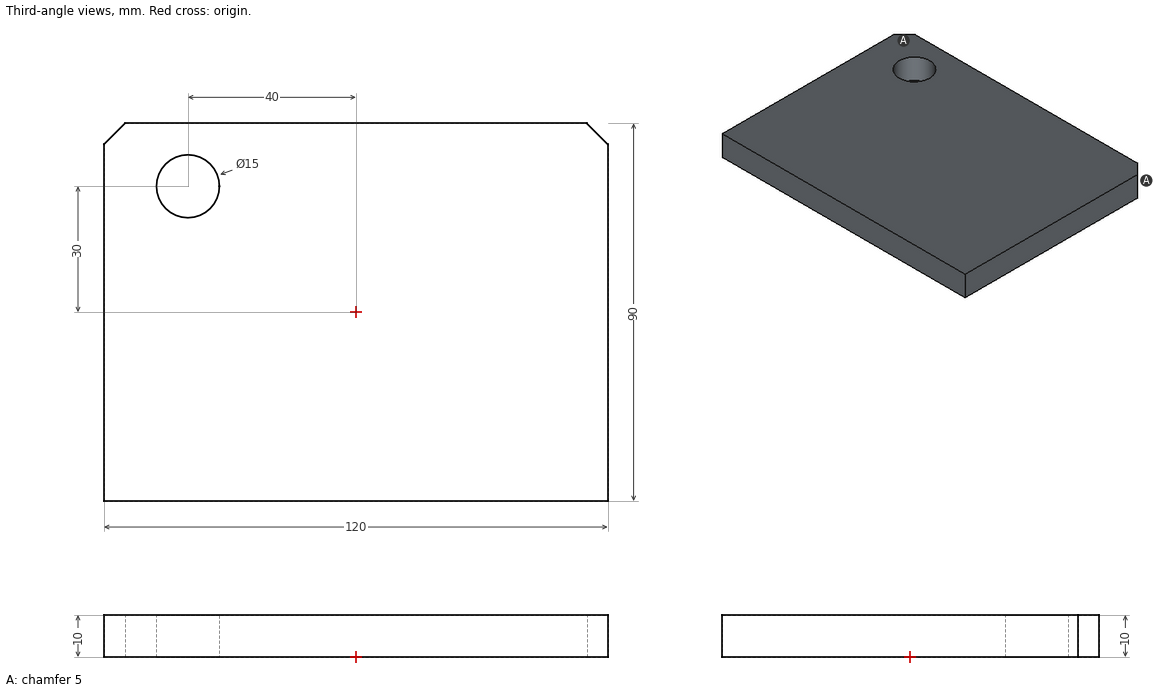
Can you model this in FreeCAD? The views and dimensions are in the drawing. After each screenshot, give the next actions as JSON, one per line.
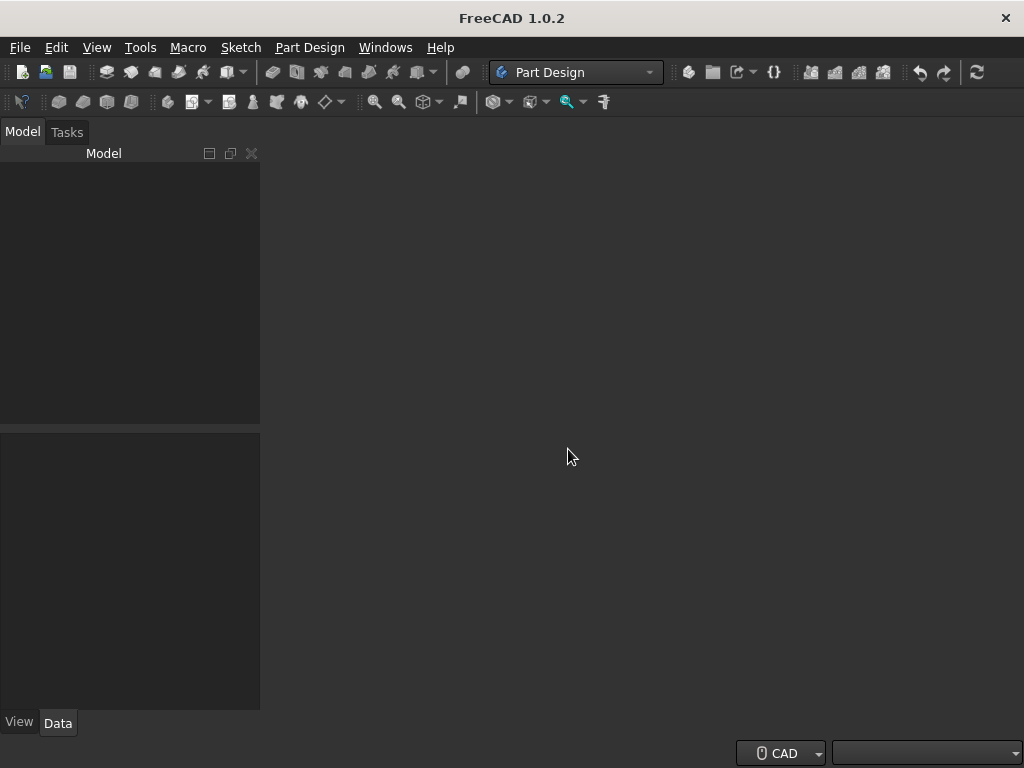
{"action": "left_click", "coordinate": [22, 72]}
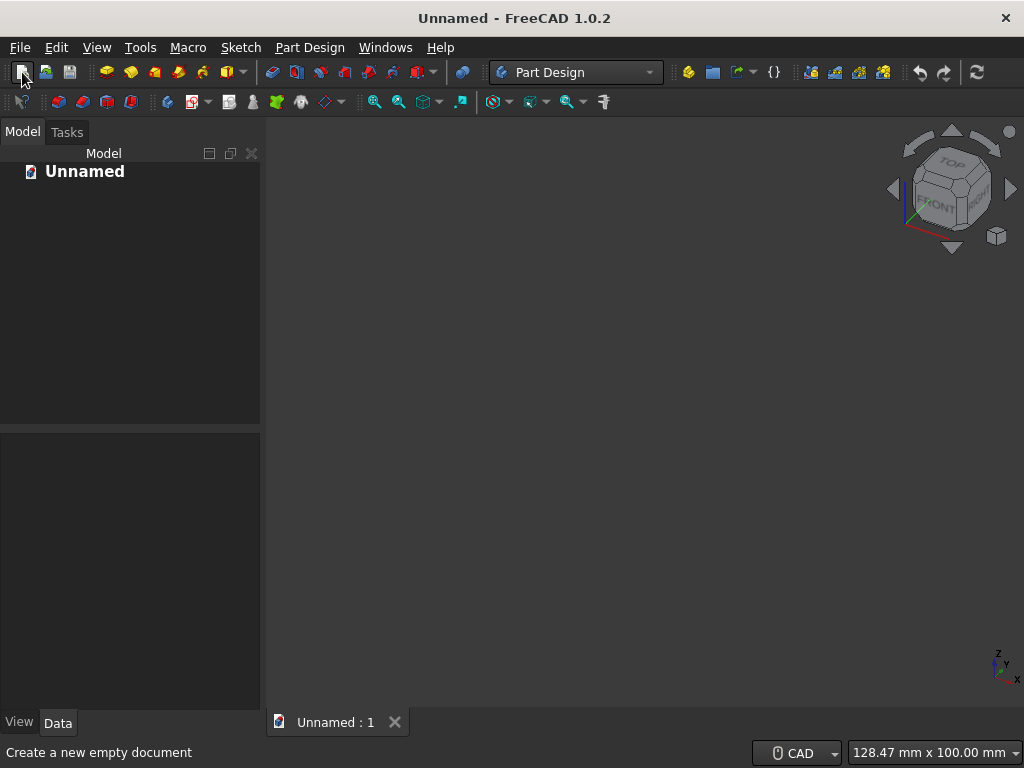
{"action": "left_click", "coordinate": [192, 102]}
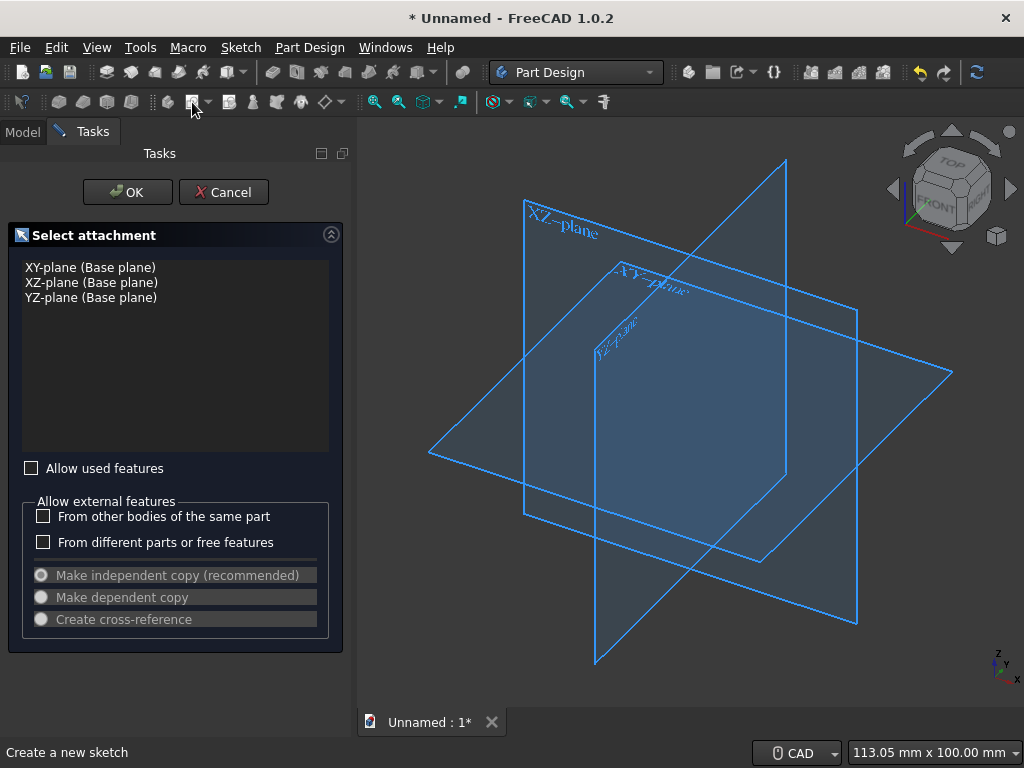
{"action": "left_click", "coordinate": [82, 268]}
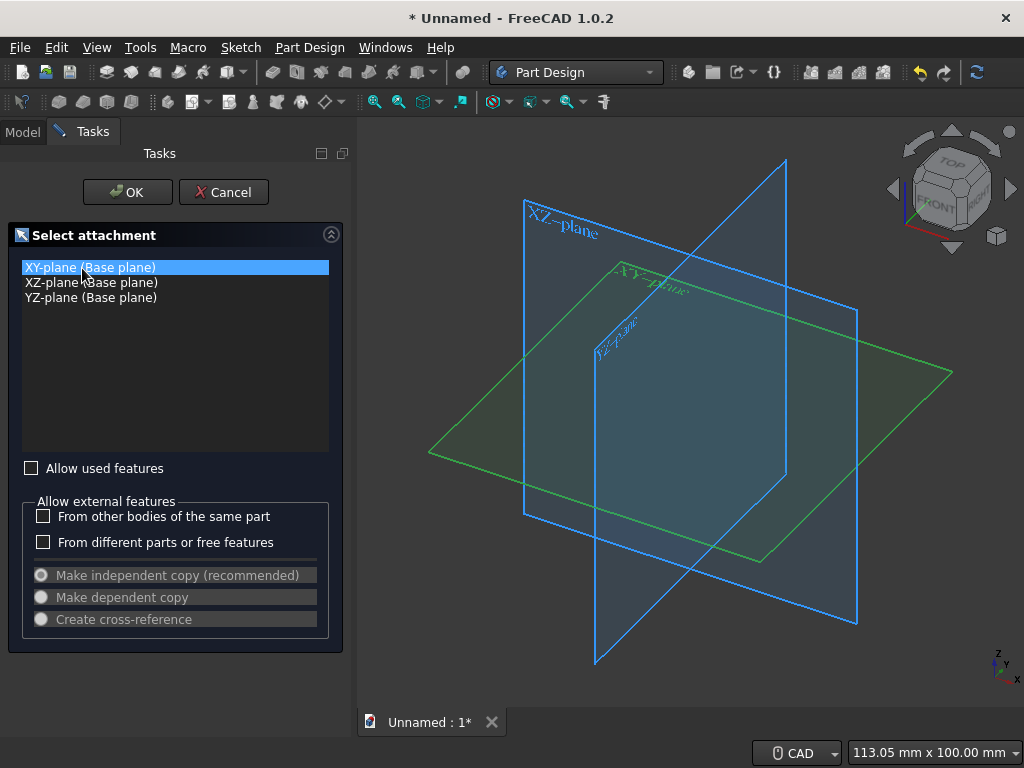
{"action": "left_click", "coordinate": [128, 192]}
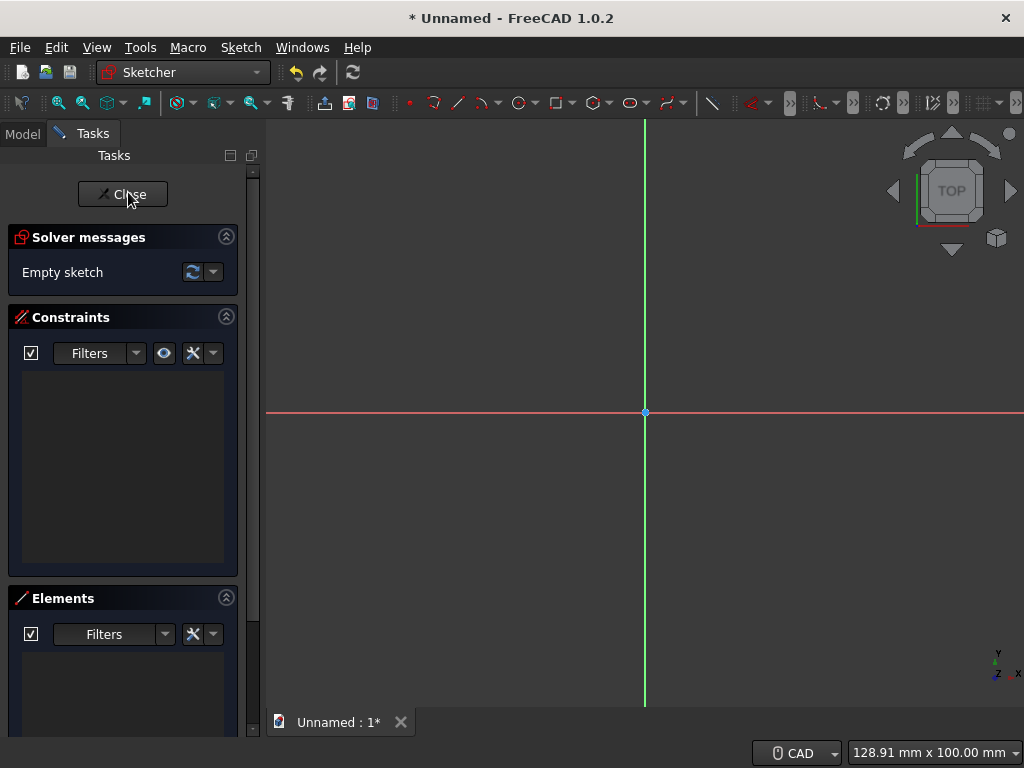
{"action": "scroll", "coordinate": [493, 413], "scroll_direction": "down", "scroll_amount": 3}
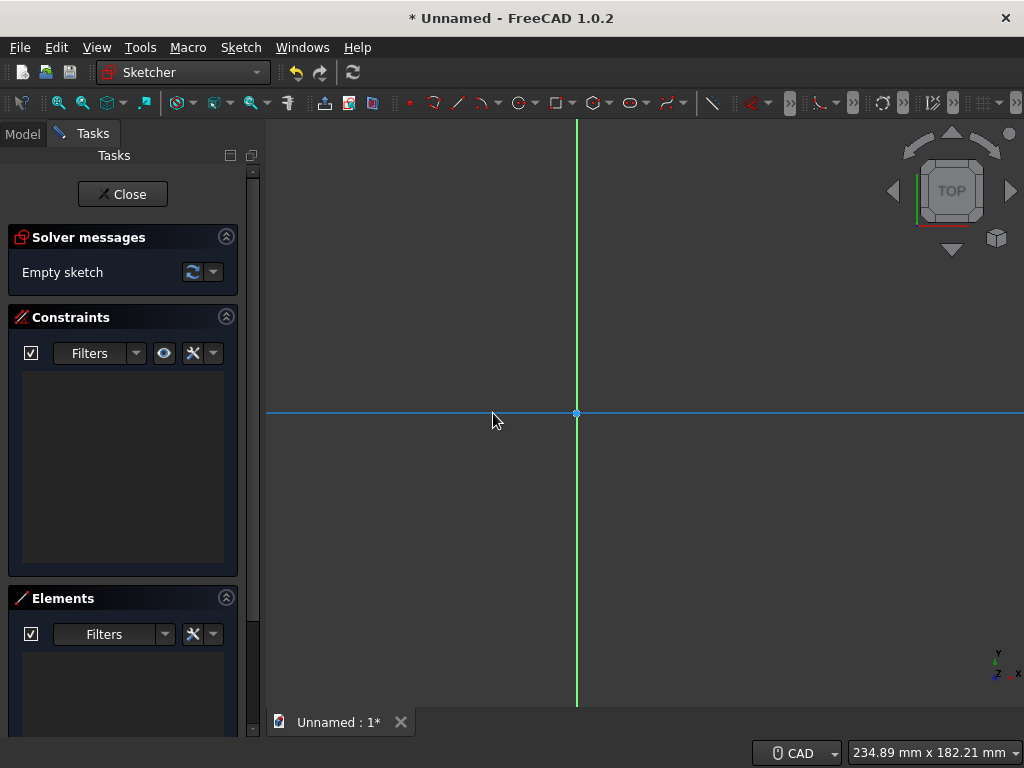
{"action": "left_click", "coordinate": [574, 104]}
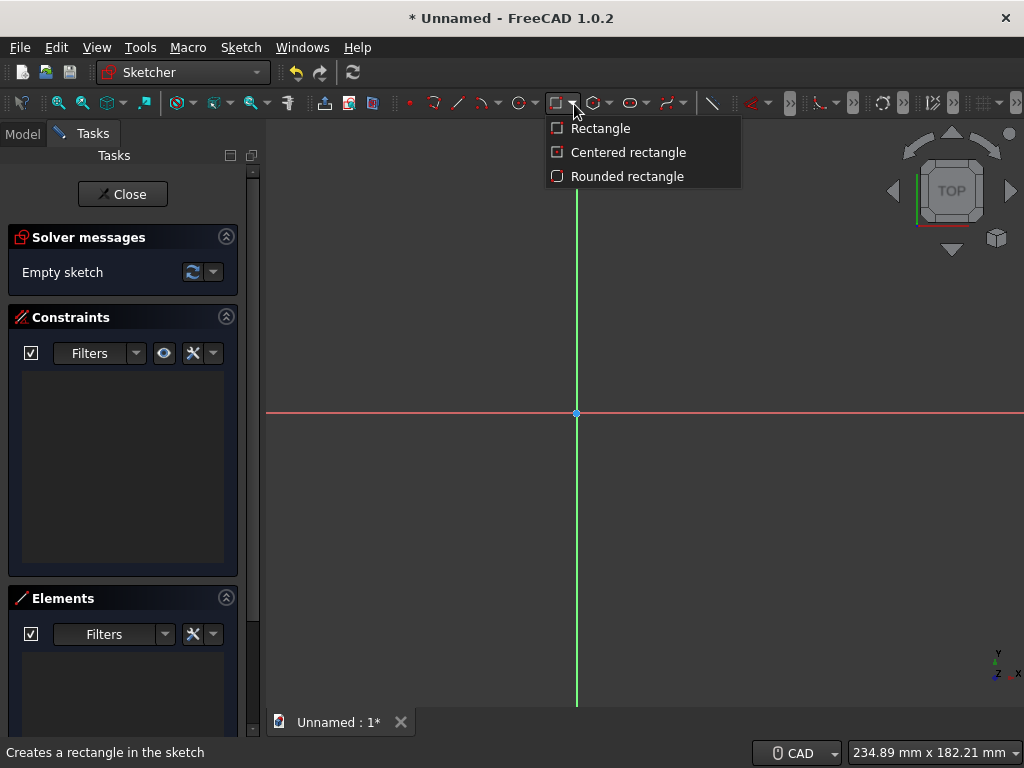
{"action": "left_click", "coordinate": [644, 152]}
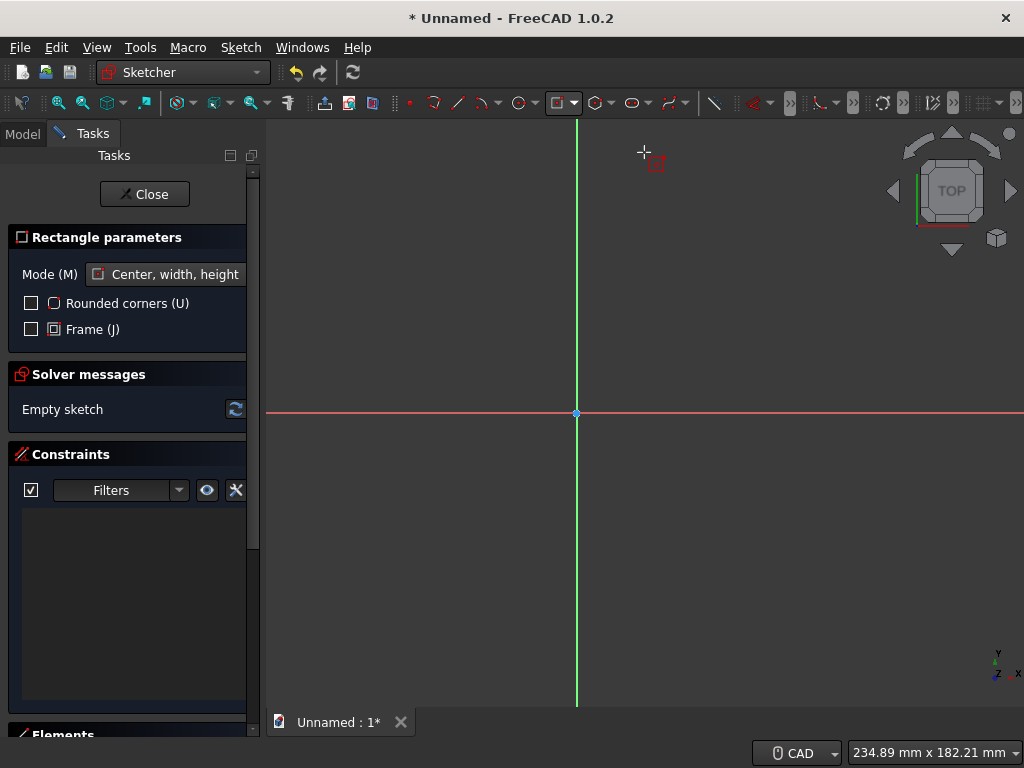
{"action": "left_click", "coordinate": [577, 413]}
{"action": "left_click", "coordinate": [770, 268]}
{"action": "key", "text": "Escape"}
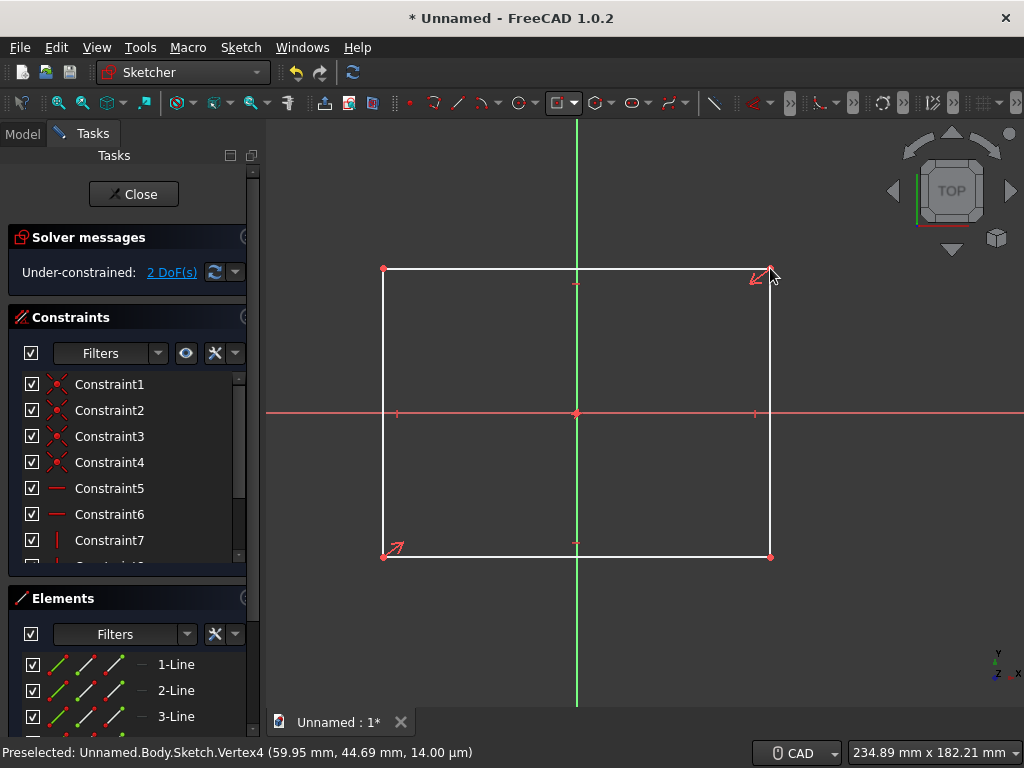
{"action": "left_click", "coordinate": [754, 104]}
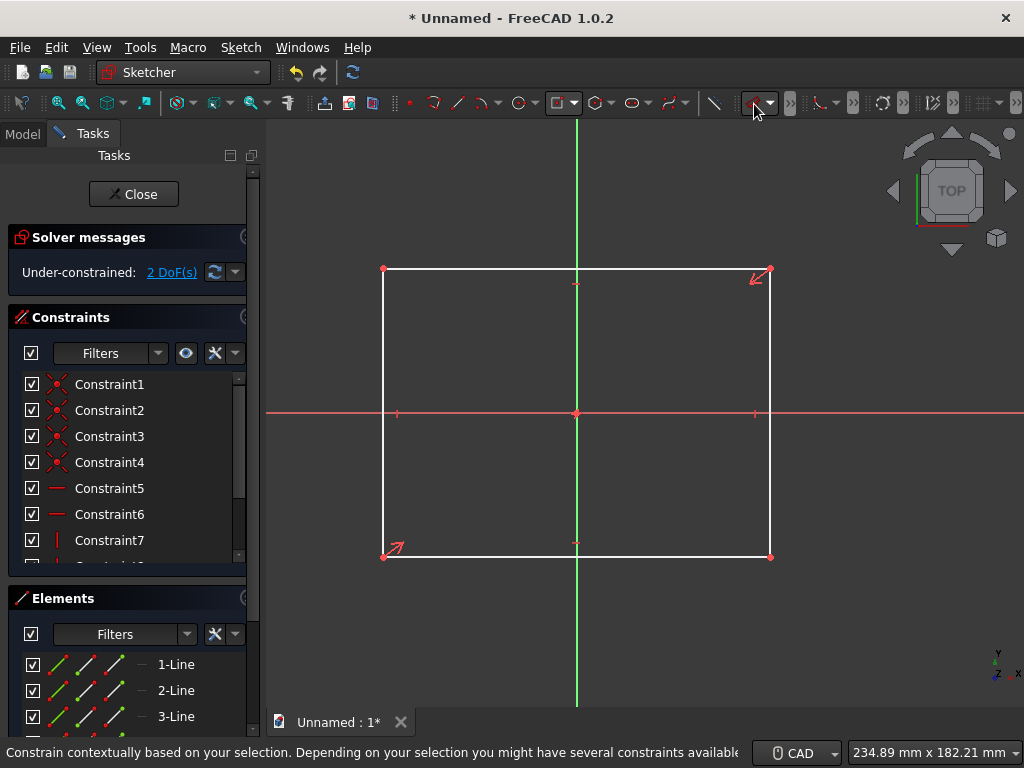
{"action": "left_click", "coordinate": [770, 471]}
{"action": "left_click", "coordinate": [804, 347]}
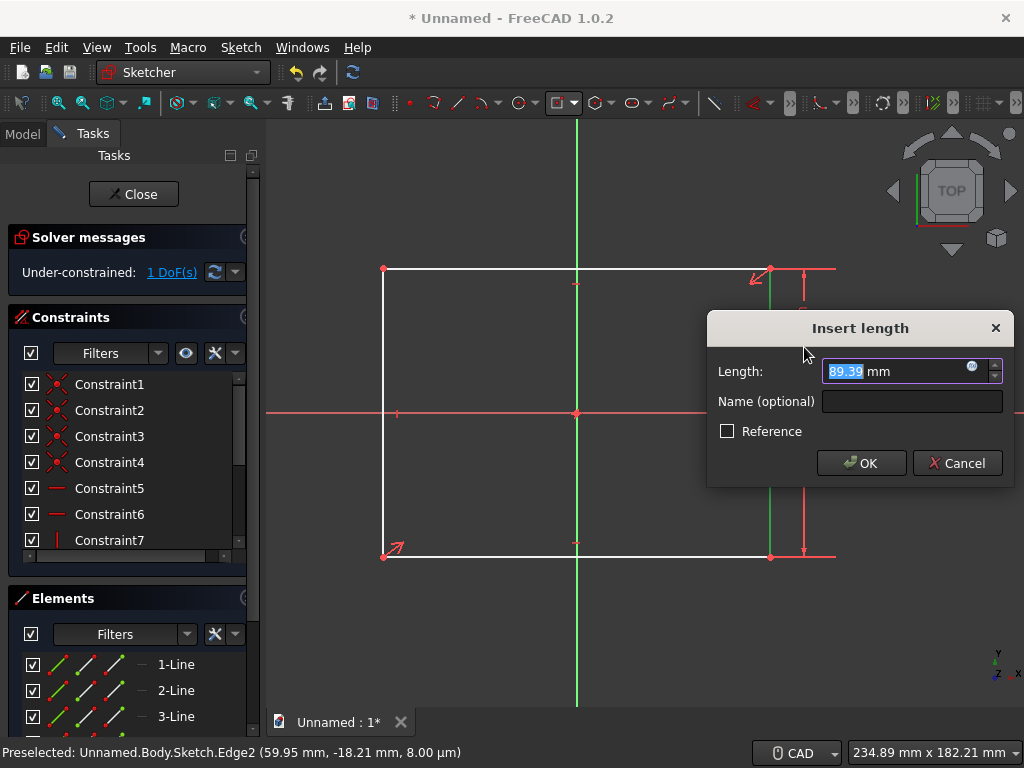
{"action": "type", "text": "90"}
{"action": "key", "text": "Return"}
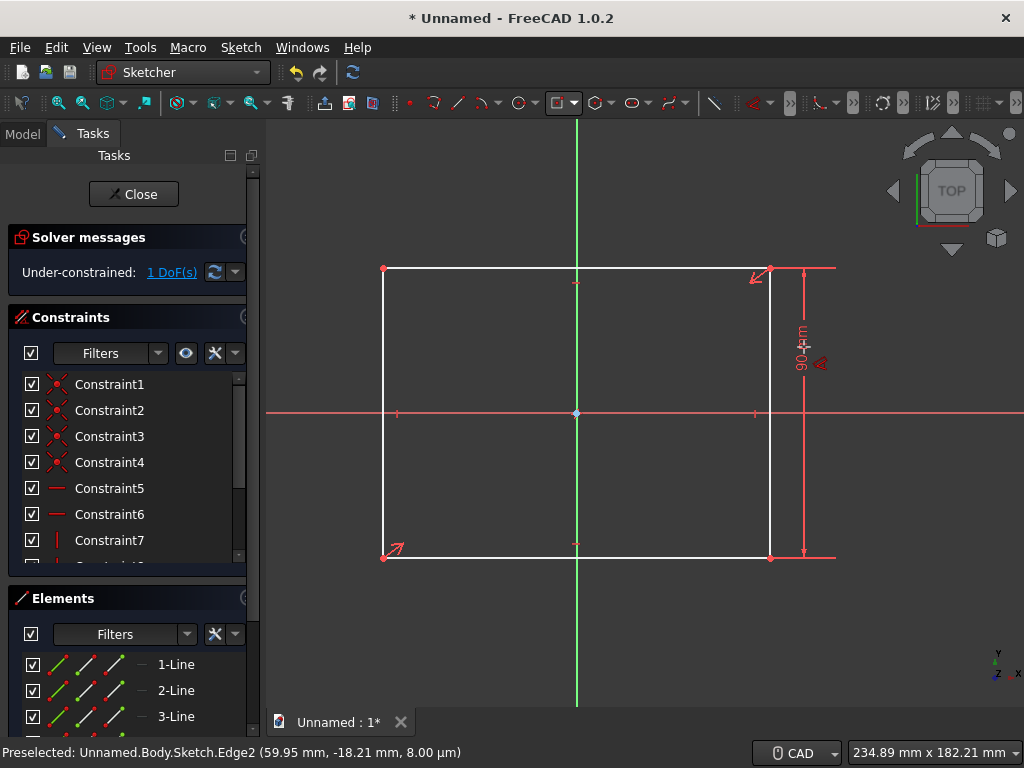
{"action": "left_click", "coordinate": [499, 558]}
{"action": "left_click", "coordinate": [488, 592]}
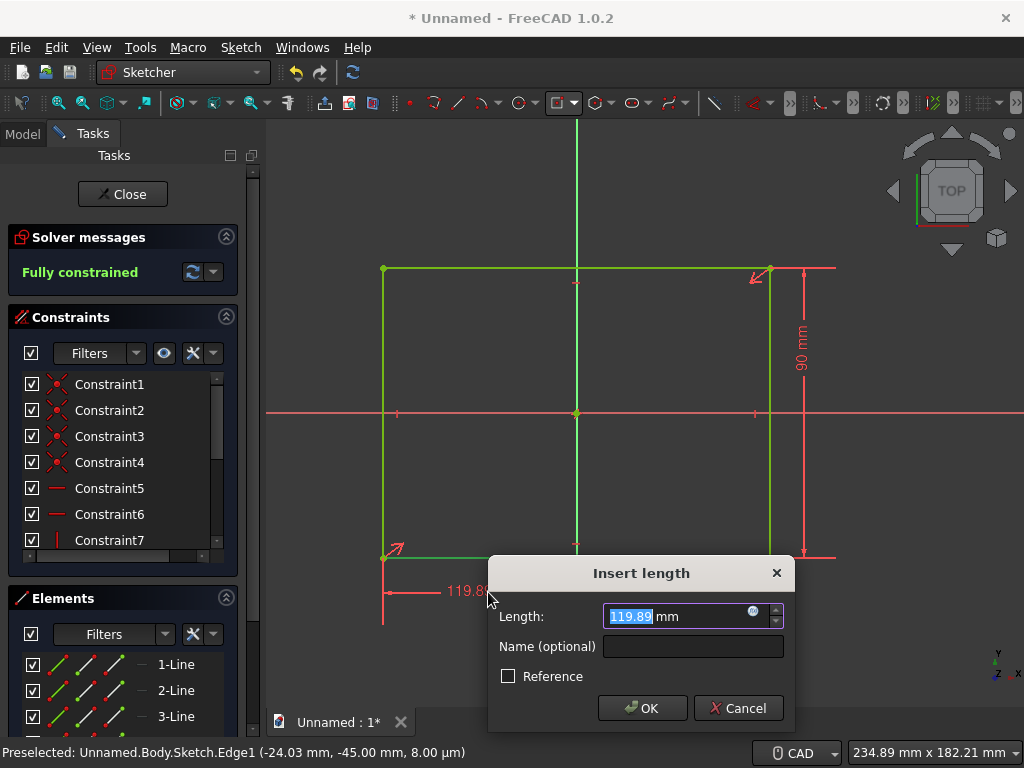
{"action": "type", "text": "120"}
{"action": "key", "text": "Return"}
{"action": "key", "text": "Escape"}